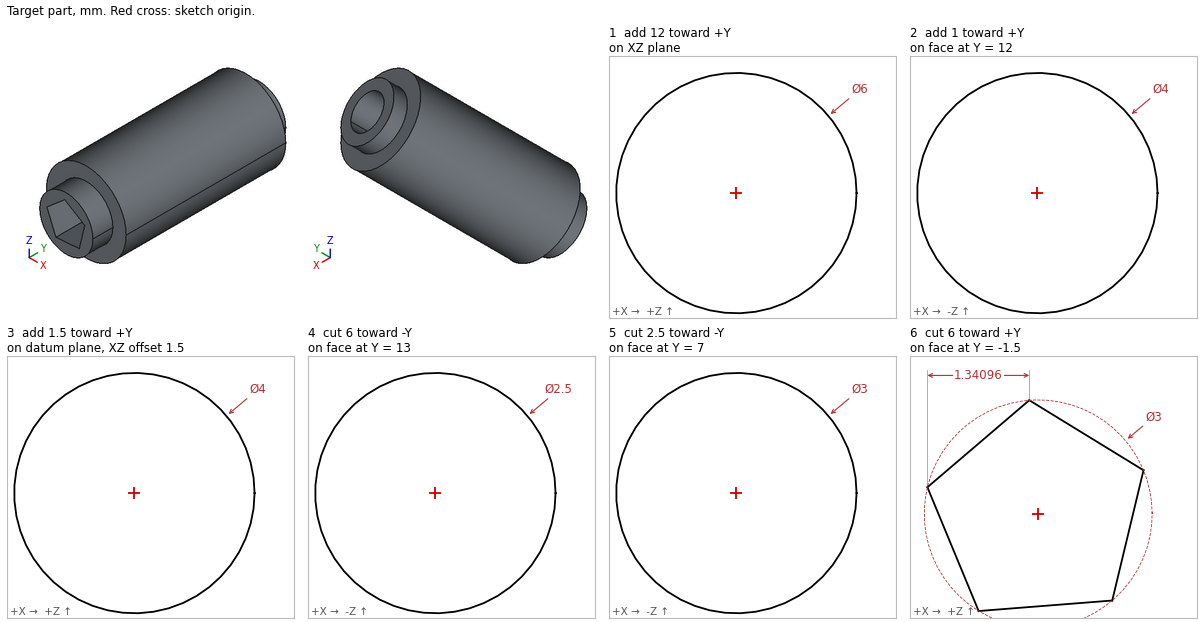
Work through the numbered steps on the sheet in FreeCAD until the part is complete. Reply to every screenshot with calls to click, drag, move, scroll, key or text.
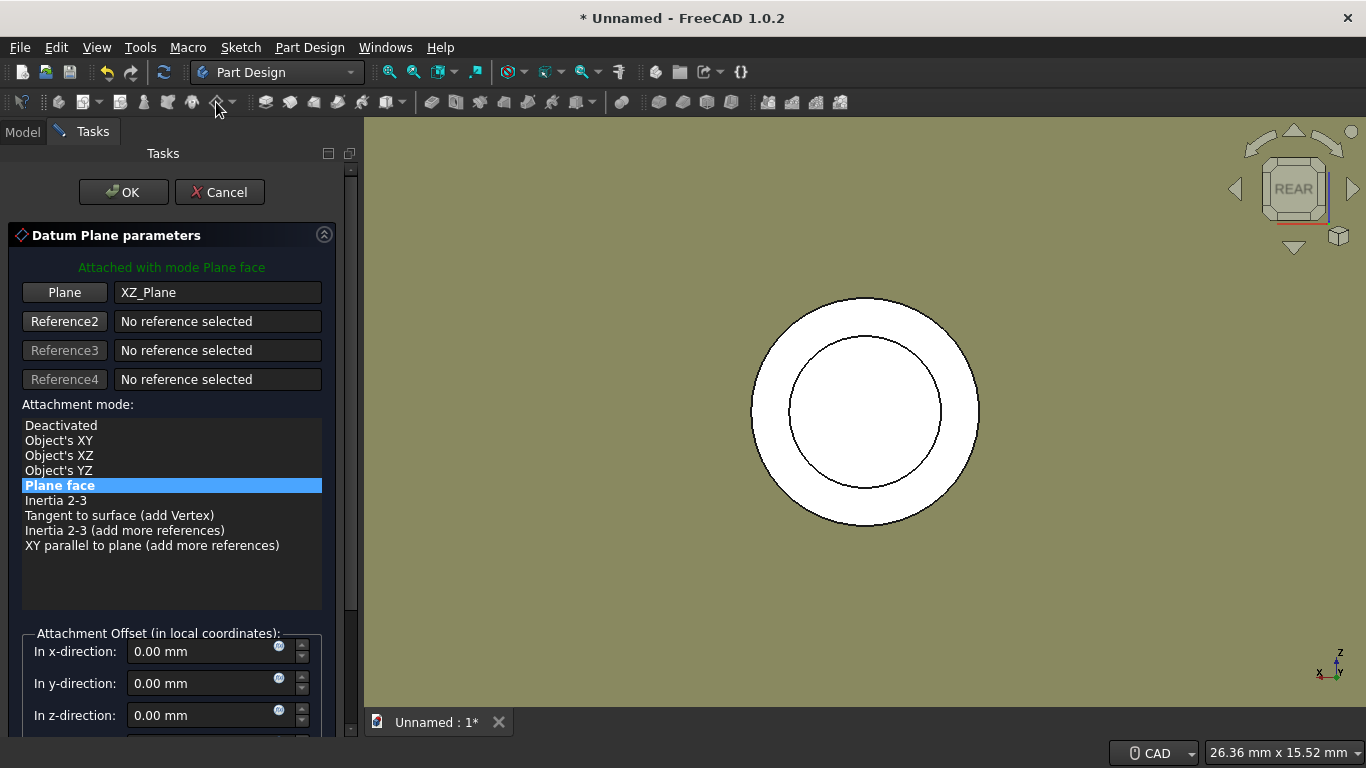
triple_click(210, 715)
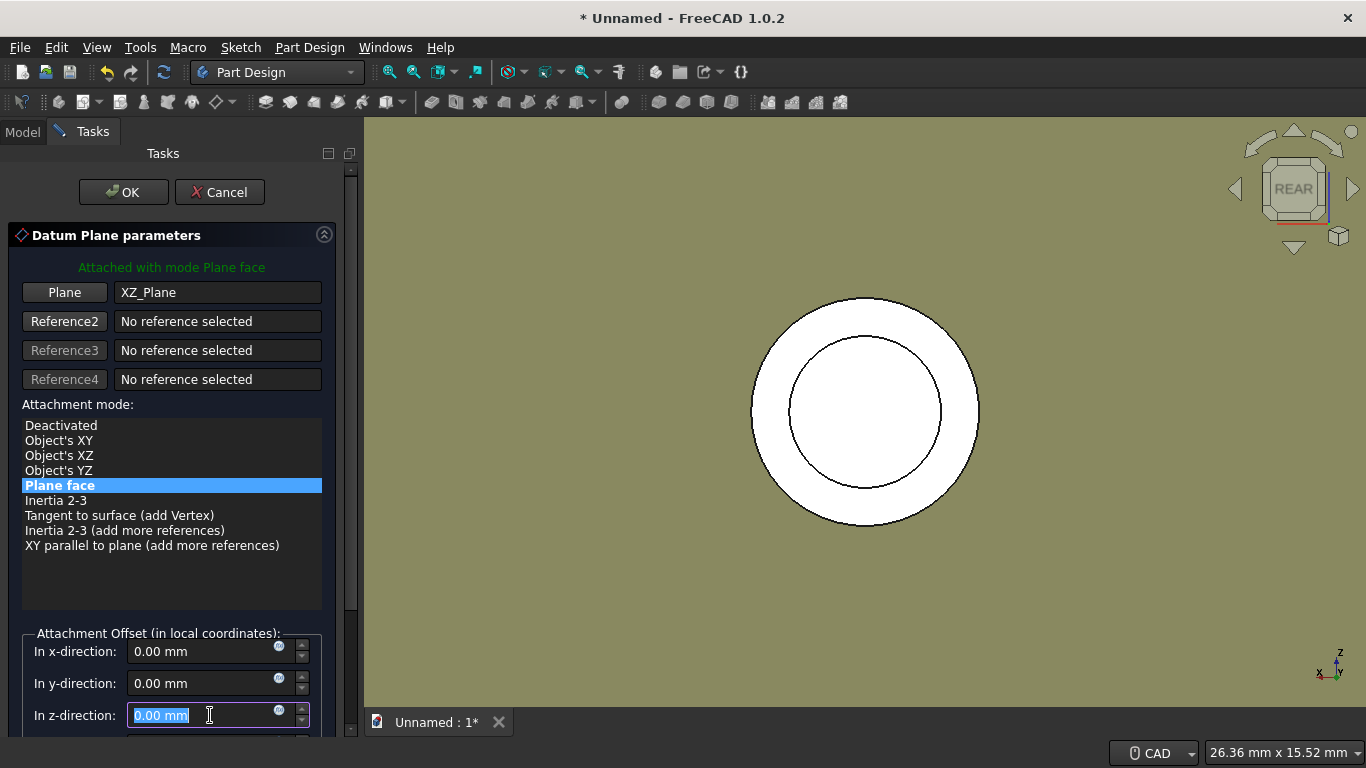
text(1.5)
key(Tab)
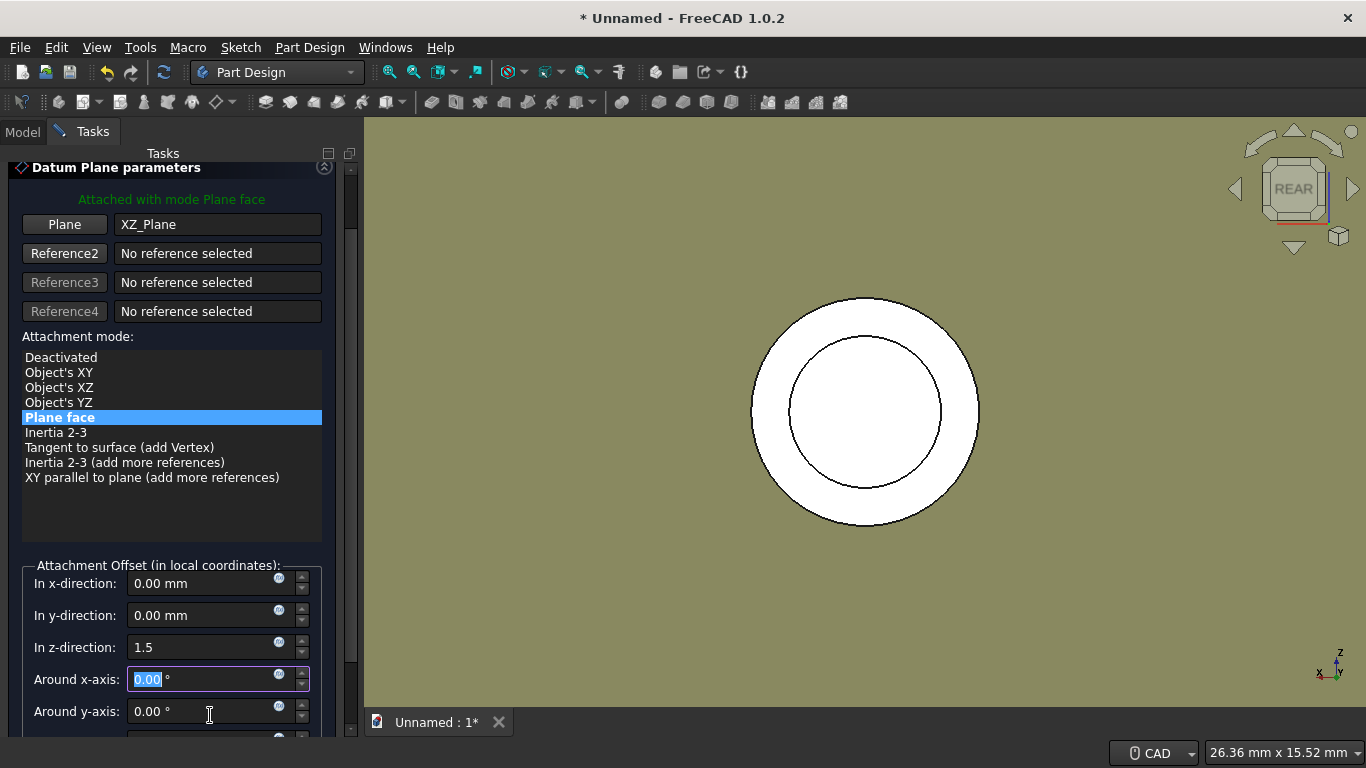
scroll(351, 450, up, 2)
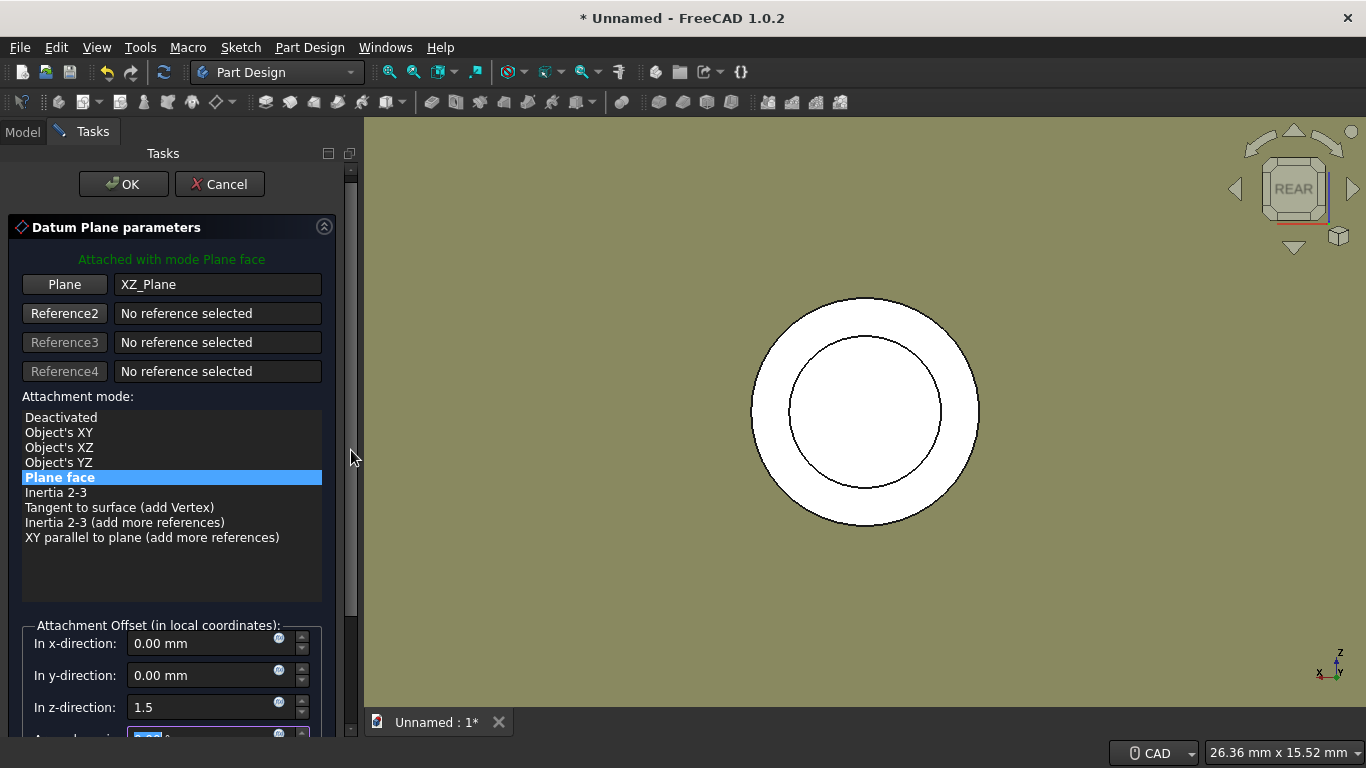
click(124, 192)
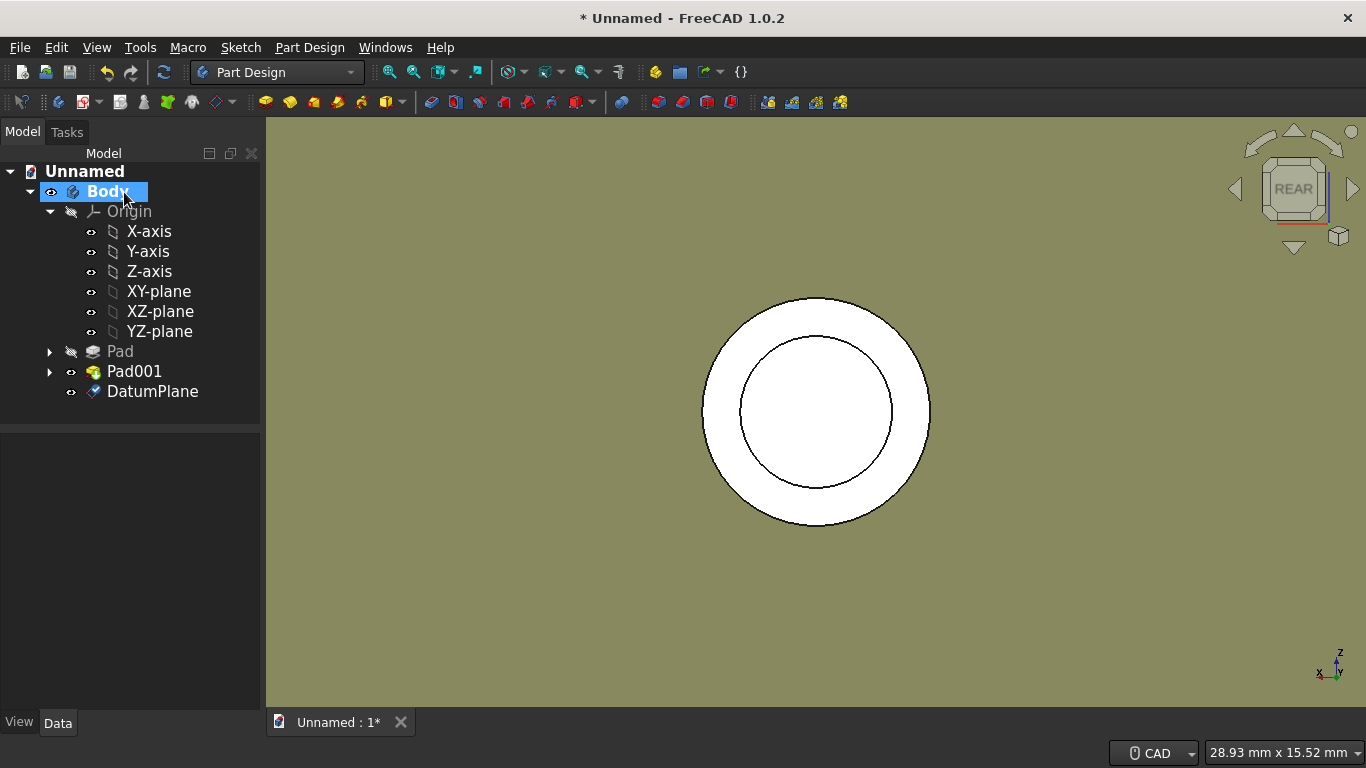
click(116, 392)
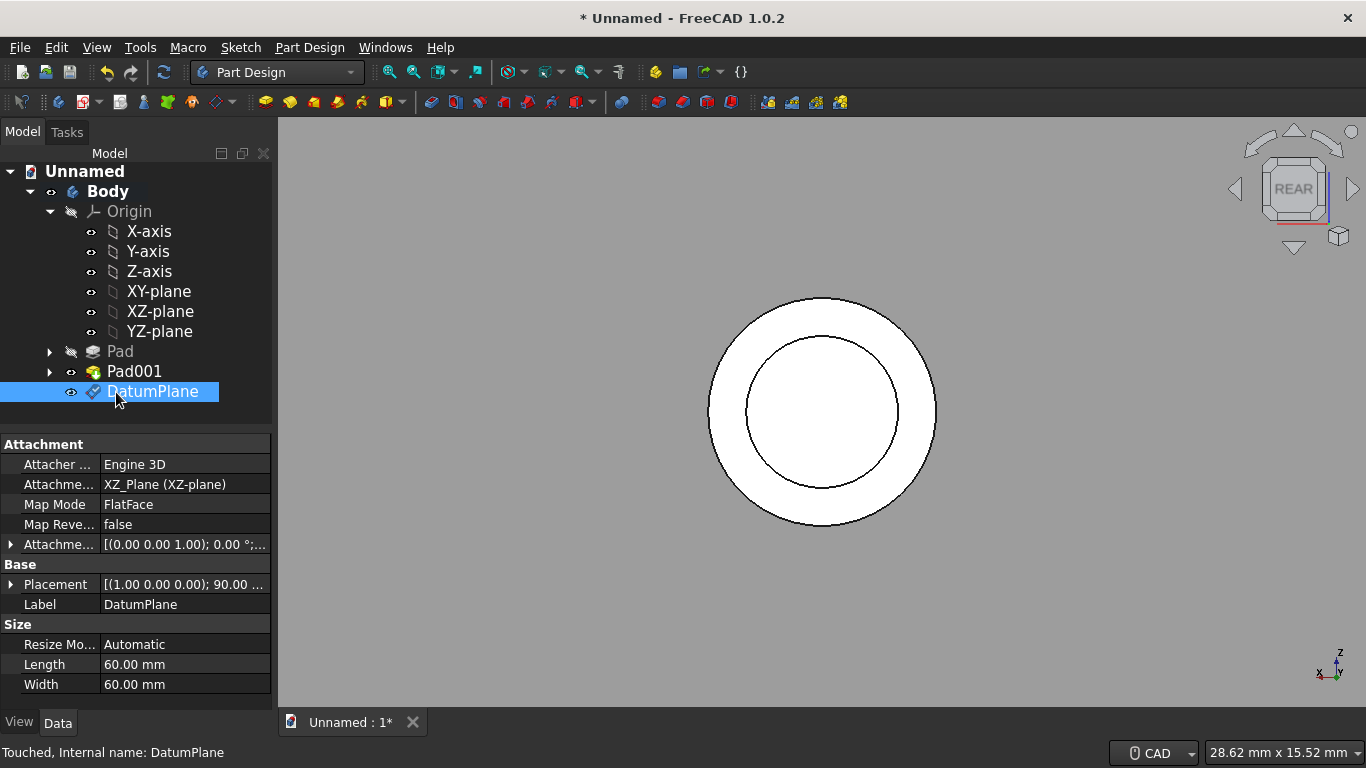
click(84, 102)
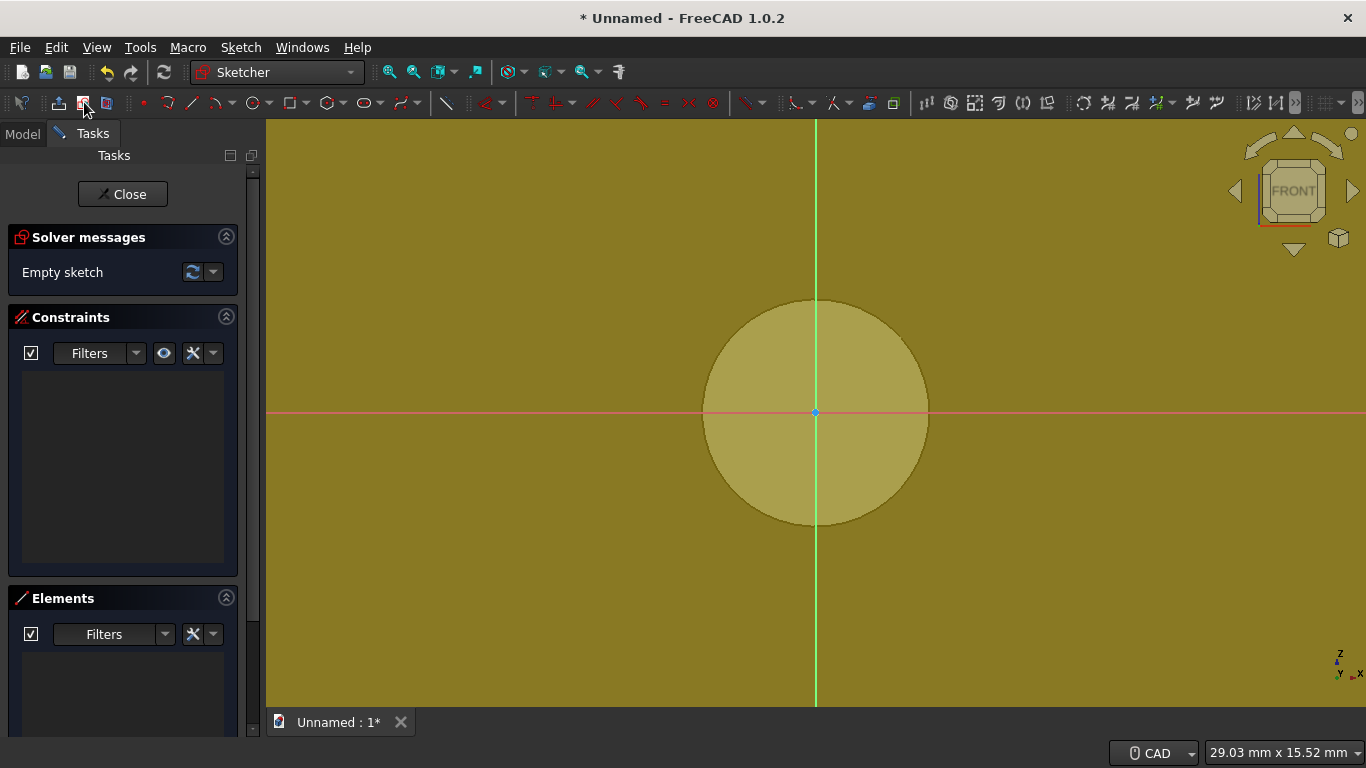
scroll(856, 413, up, 5)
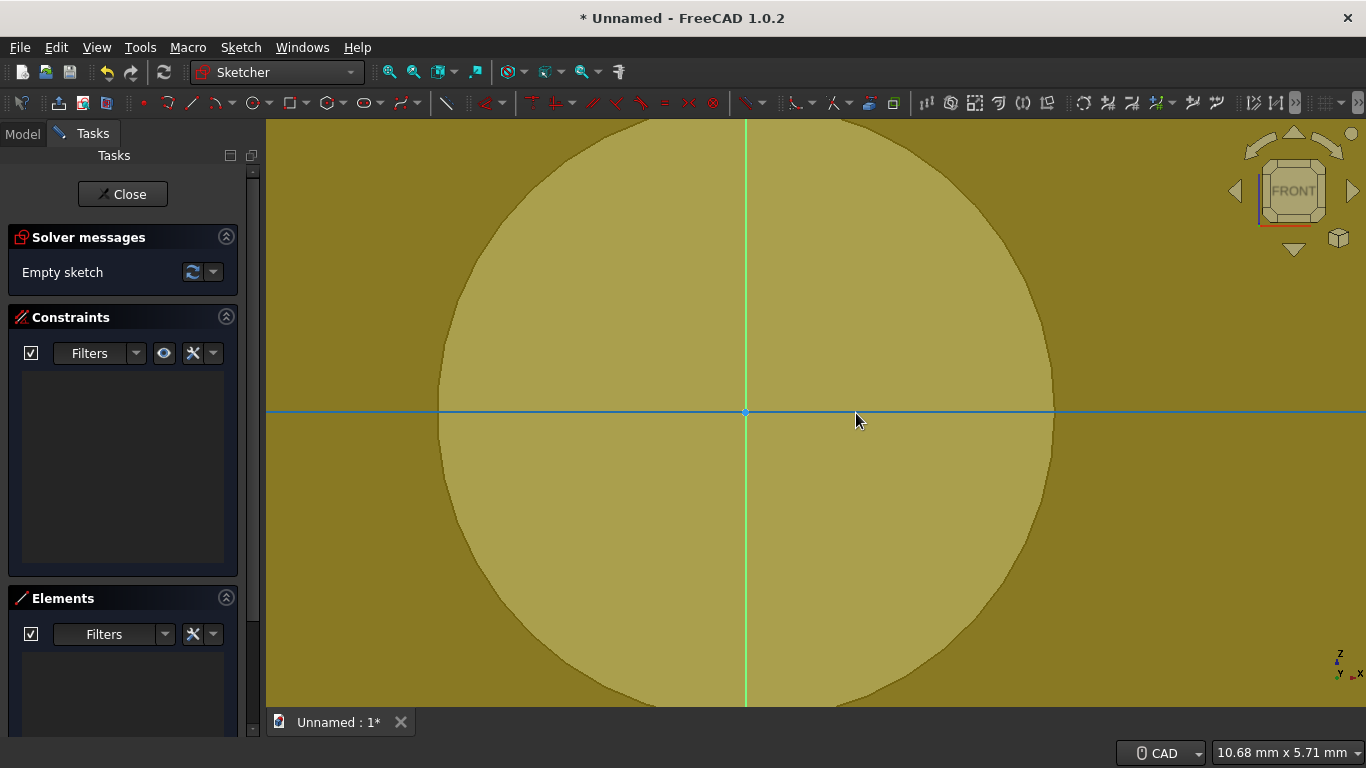
click(254, 104)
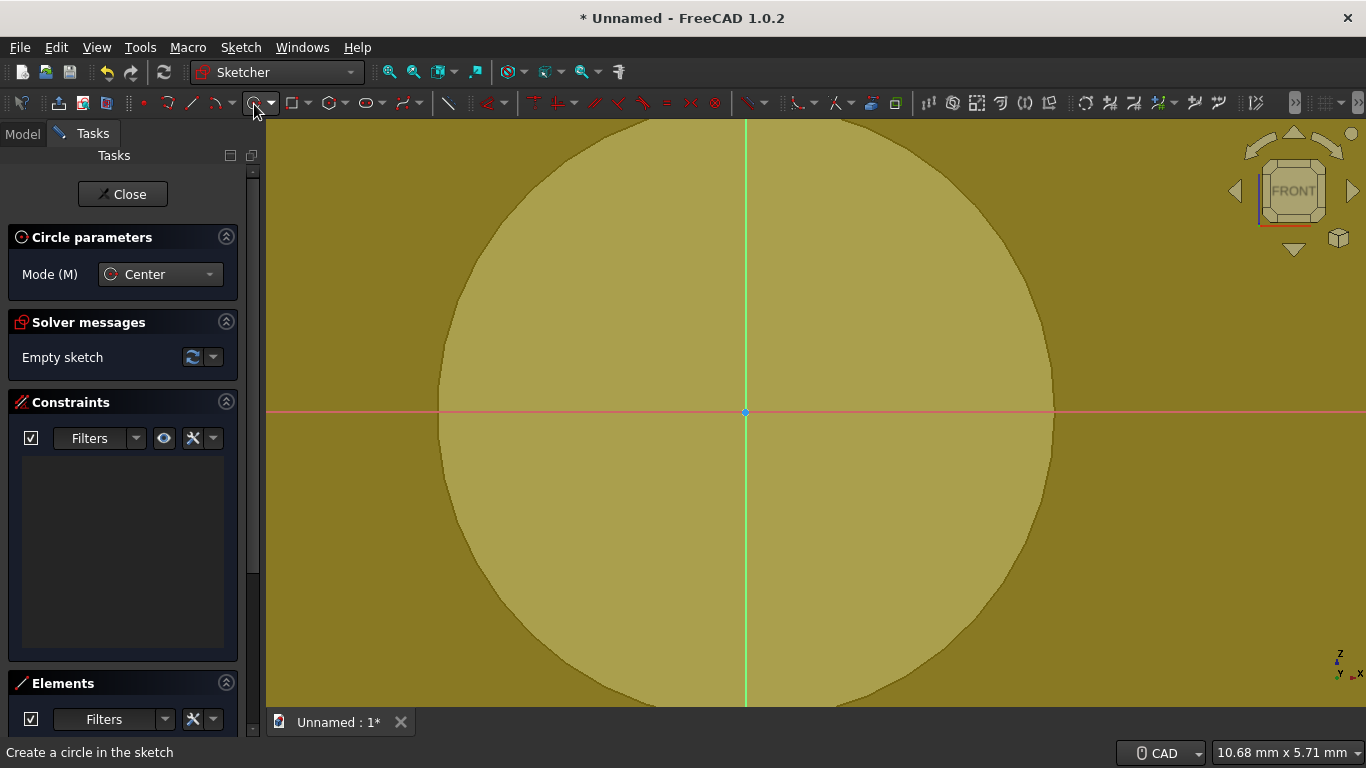
click(746, 412)
move(892, 266)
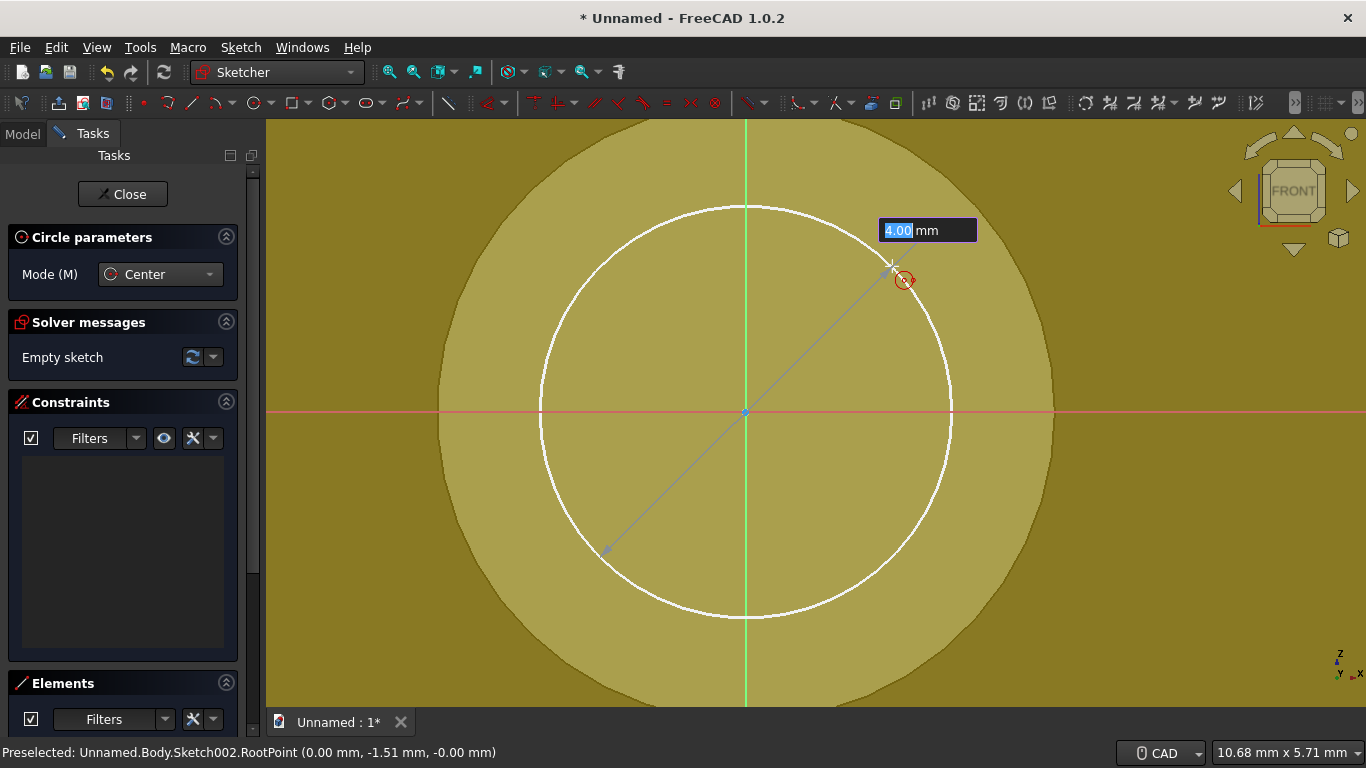
text(4)
key(Return)
key(Escape)